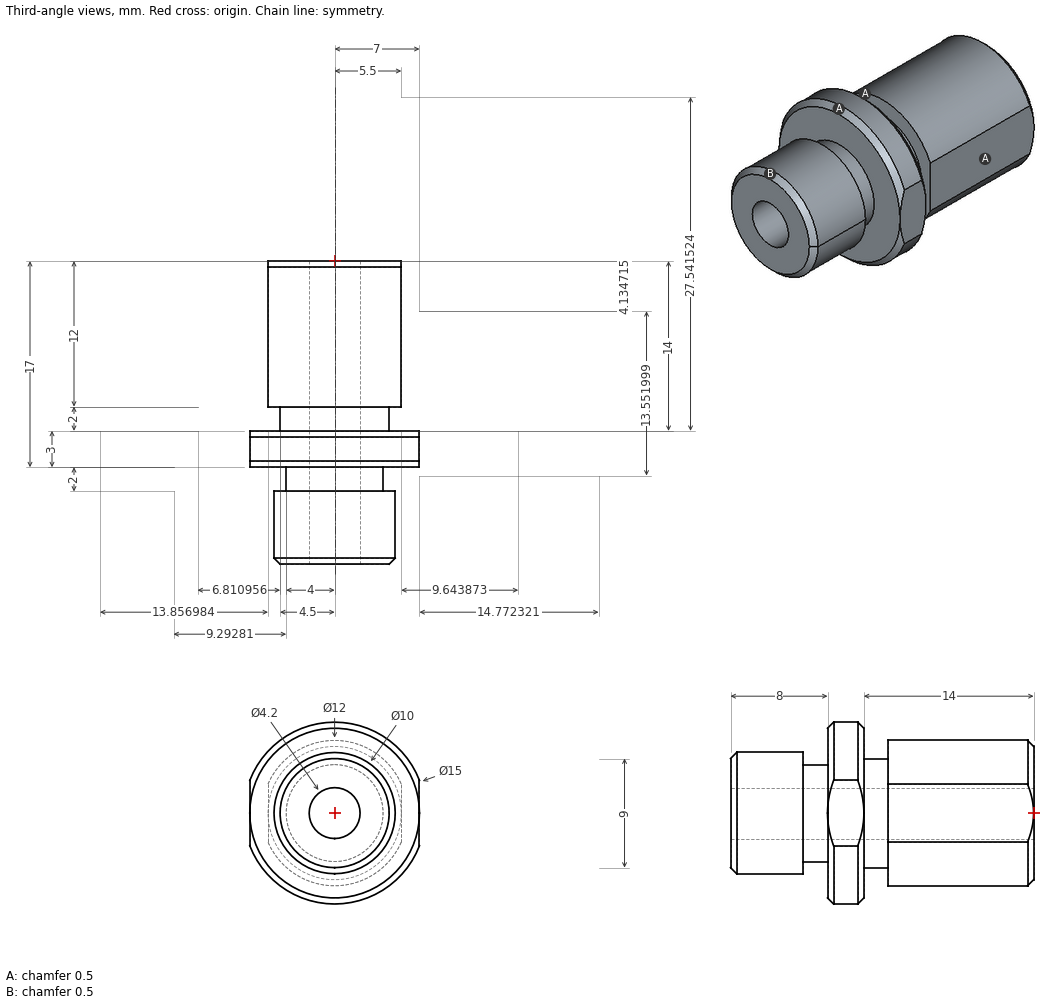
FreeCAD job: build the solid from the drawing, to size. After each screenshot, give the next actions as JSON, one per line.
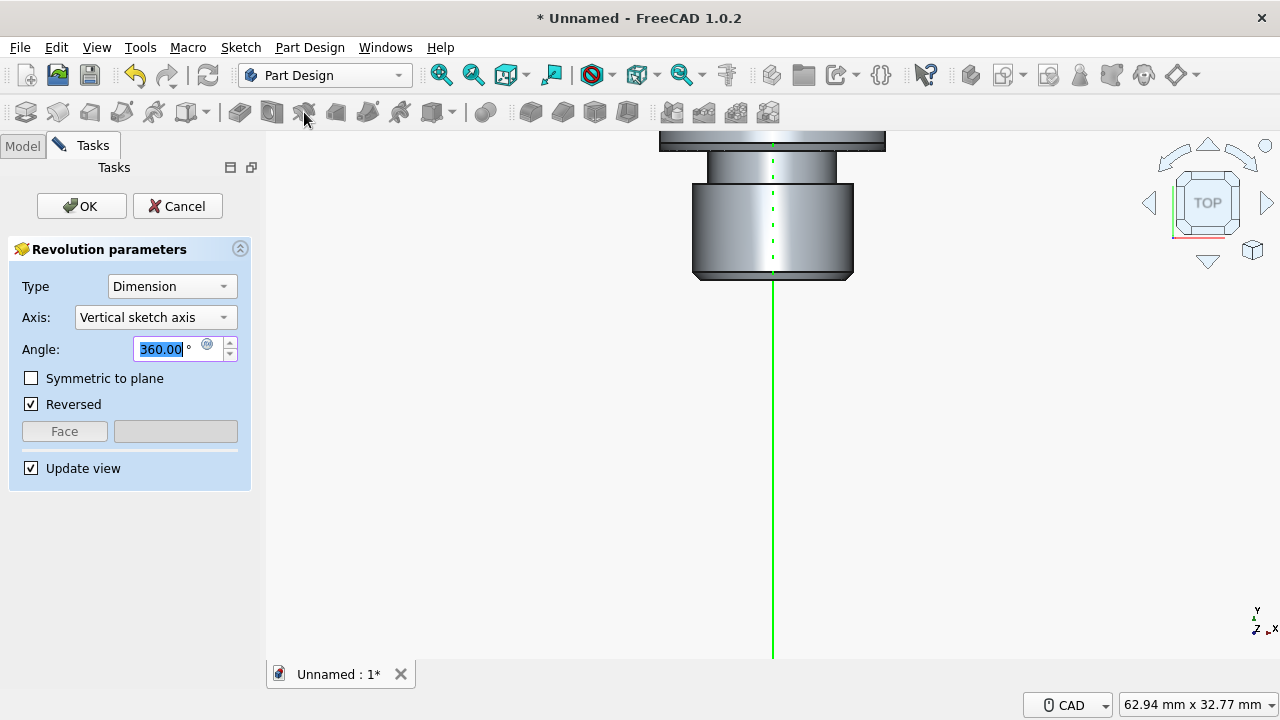
{"action": "left_click", "coordinate": [82, 206]}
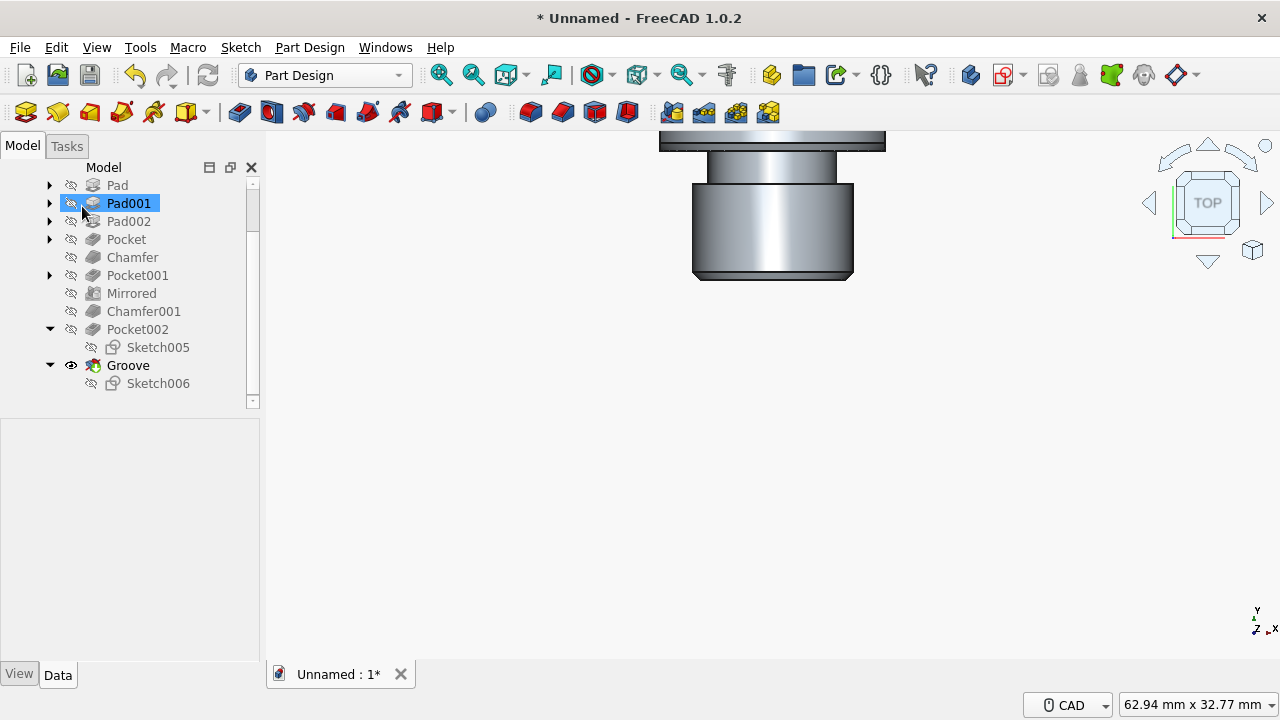
{"action": "key", "text": "v f"}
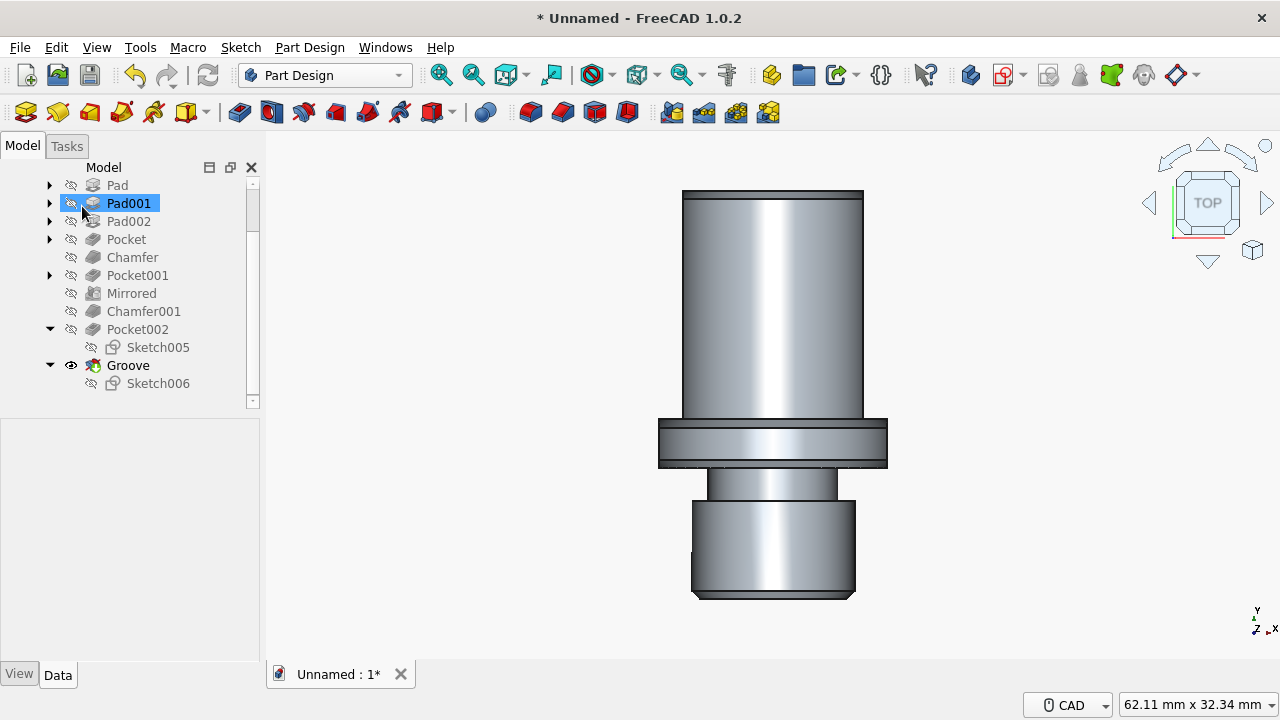
{"action": "left_click", "coordinate": [1004, 76]}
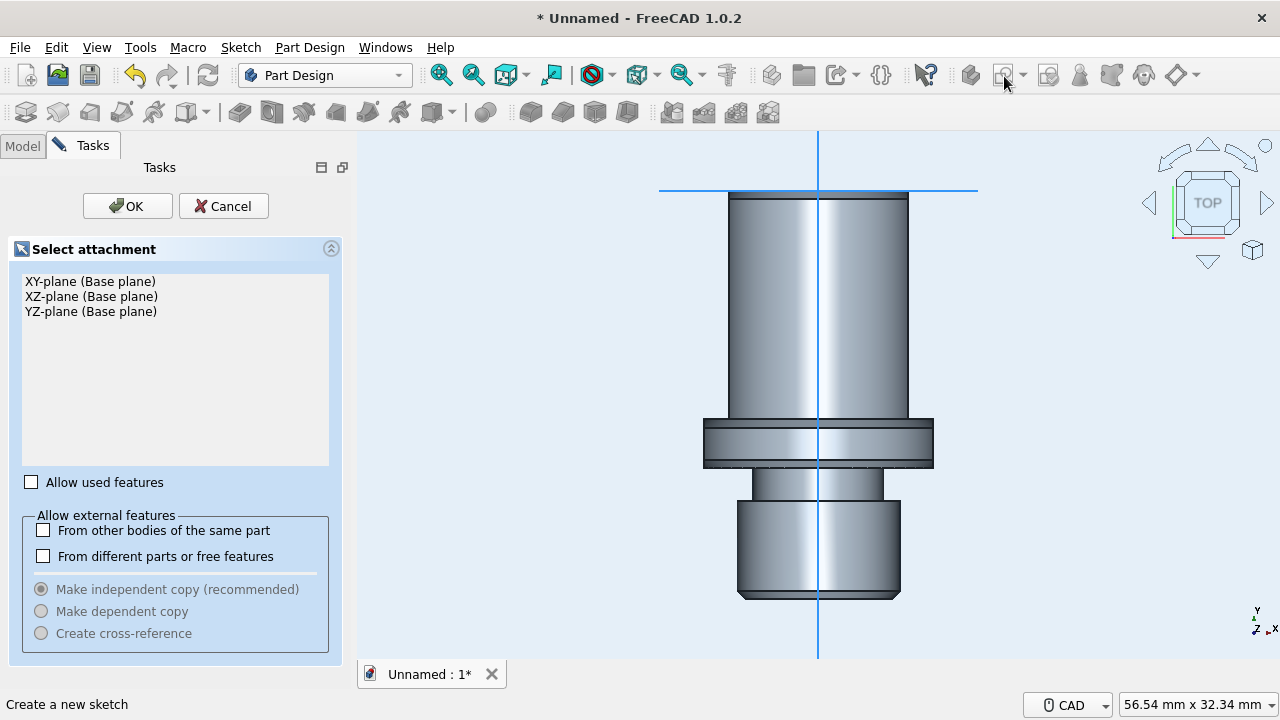
{"action": "left_click", "coordinate": [82, 282]}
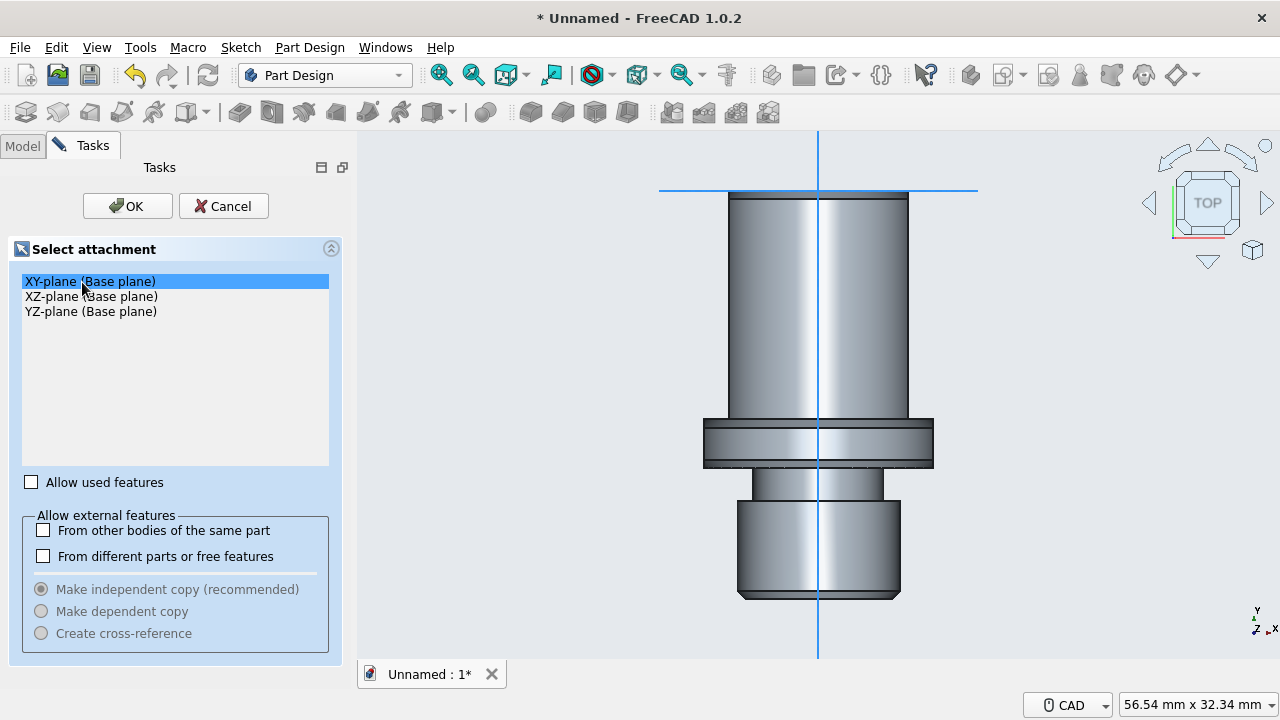
{"action": "left_click", "coordinate": [128, 206]}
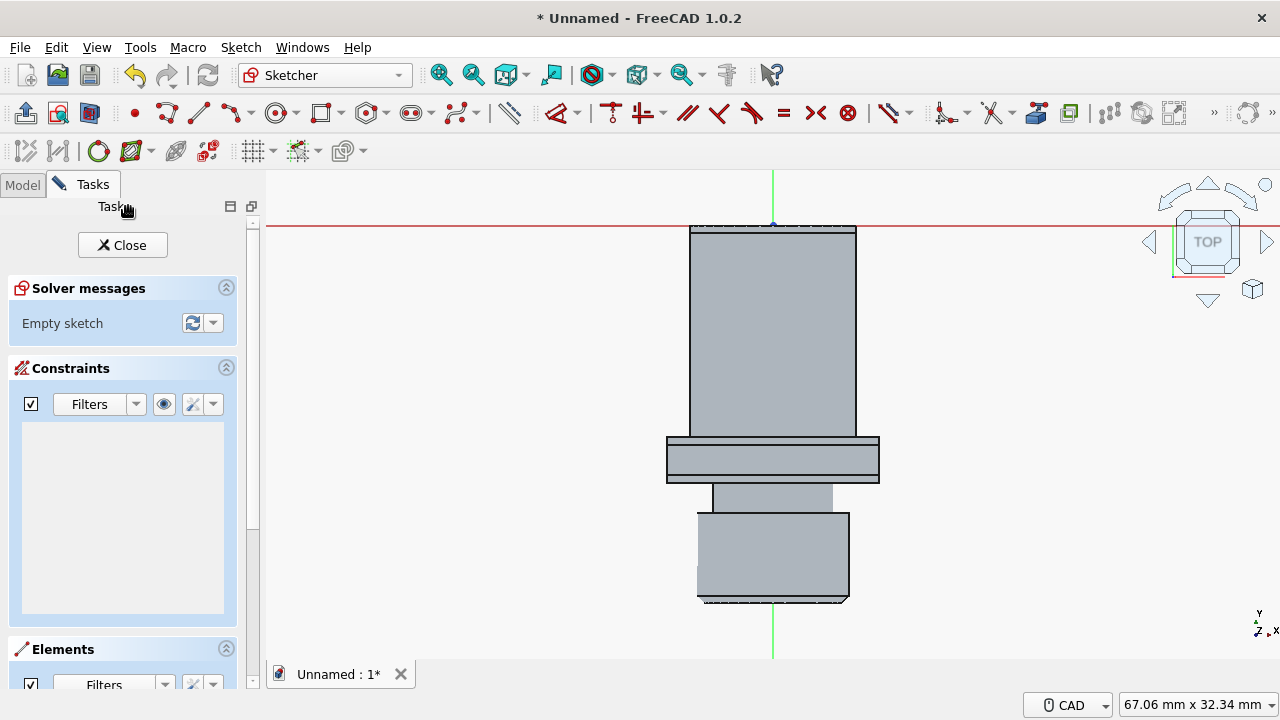
{"action": "key", "text": "q s"}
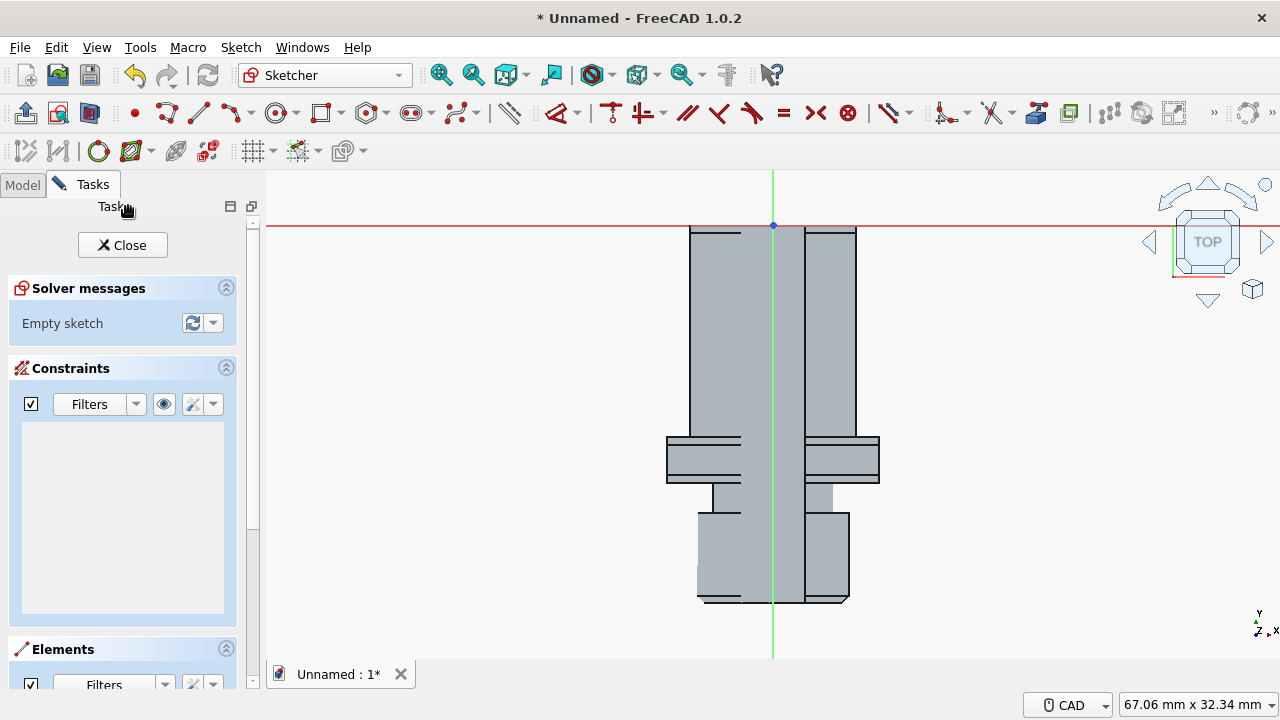
{"action": "scroll", "coordinate": [653, 198], "scroll_direction": "up", "scroll_amount": 2}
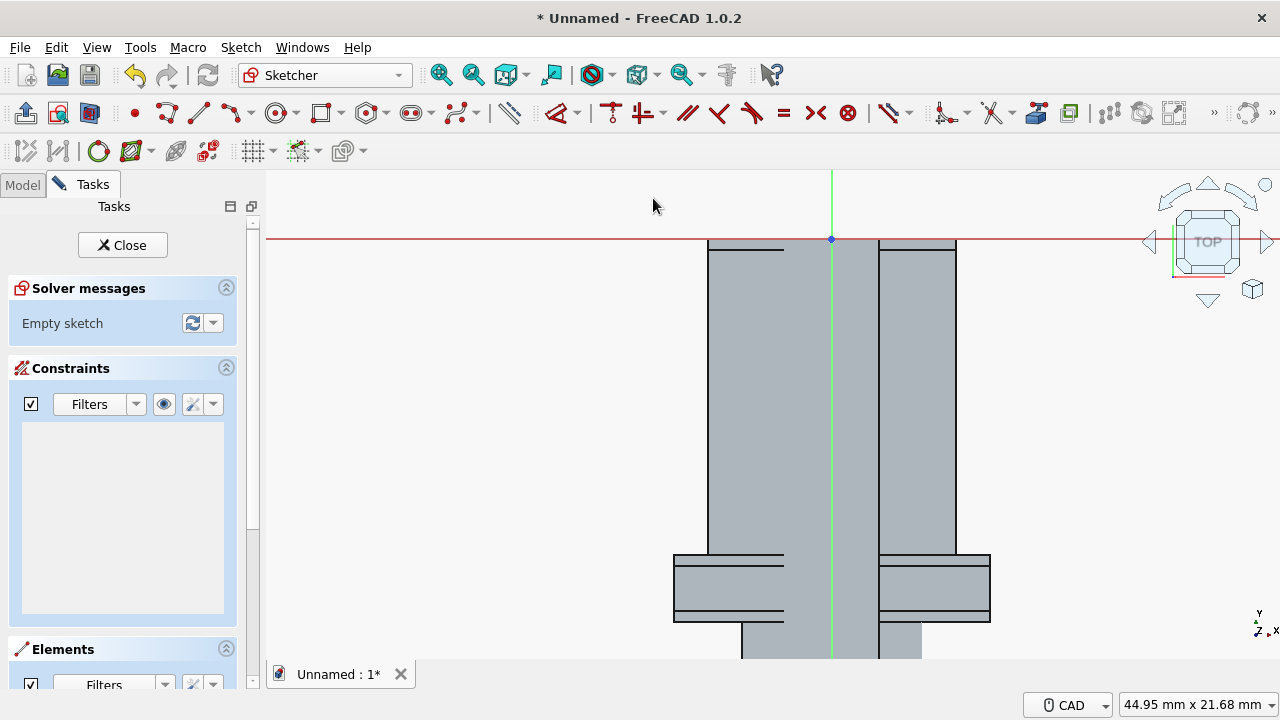
{"action": "key", "text": "g r"}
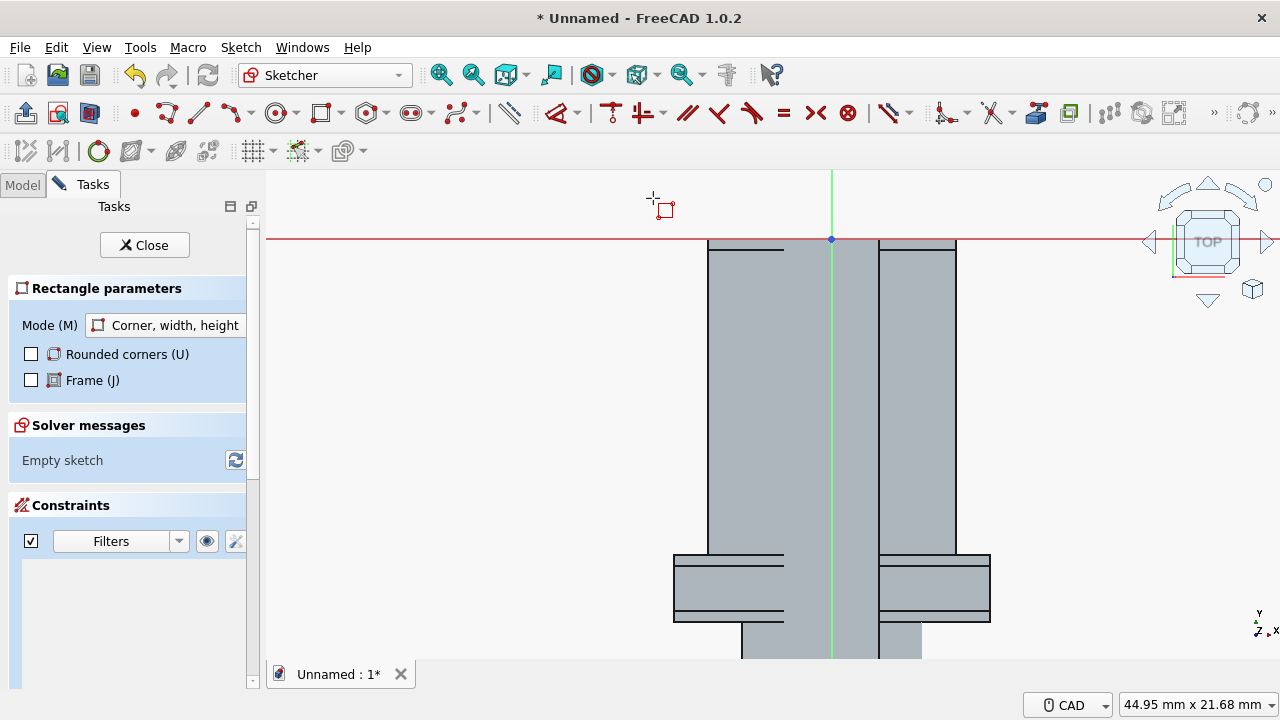
{"action": "left_click", "coordinate": [577, 510]}
{"action": "left_click", "coordinate": [730, 555]}
{"action": "key", "text": "Escape"}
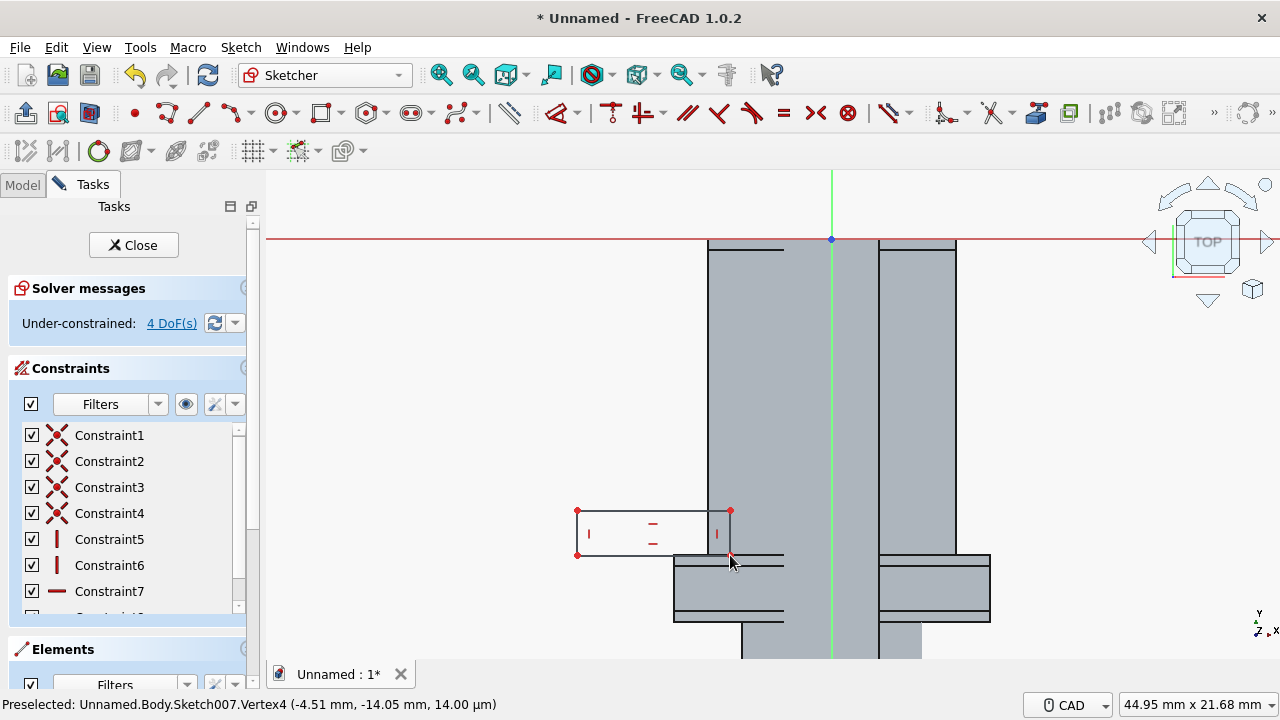
{"action": "key", "text": "d"}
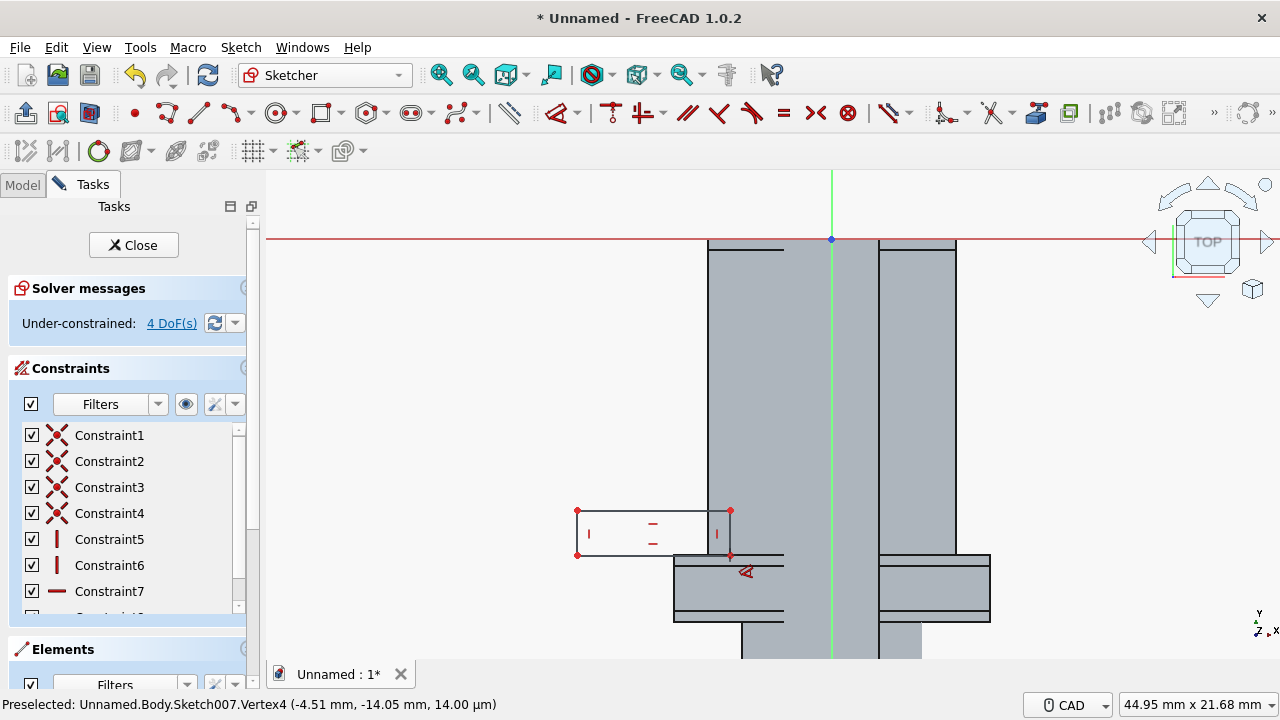
{"action": "left_click", "coordinate": [577, 525]}
{"action": "left_click", "coordinate": [543, 534]}